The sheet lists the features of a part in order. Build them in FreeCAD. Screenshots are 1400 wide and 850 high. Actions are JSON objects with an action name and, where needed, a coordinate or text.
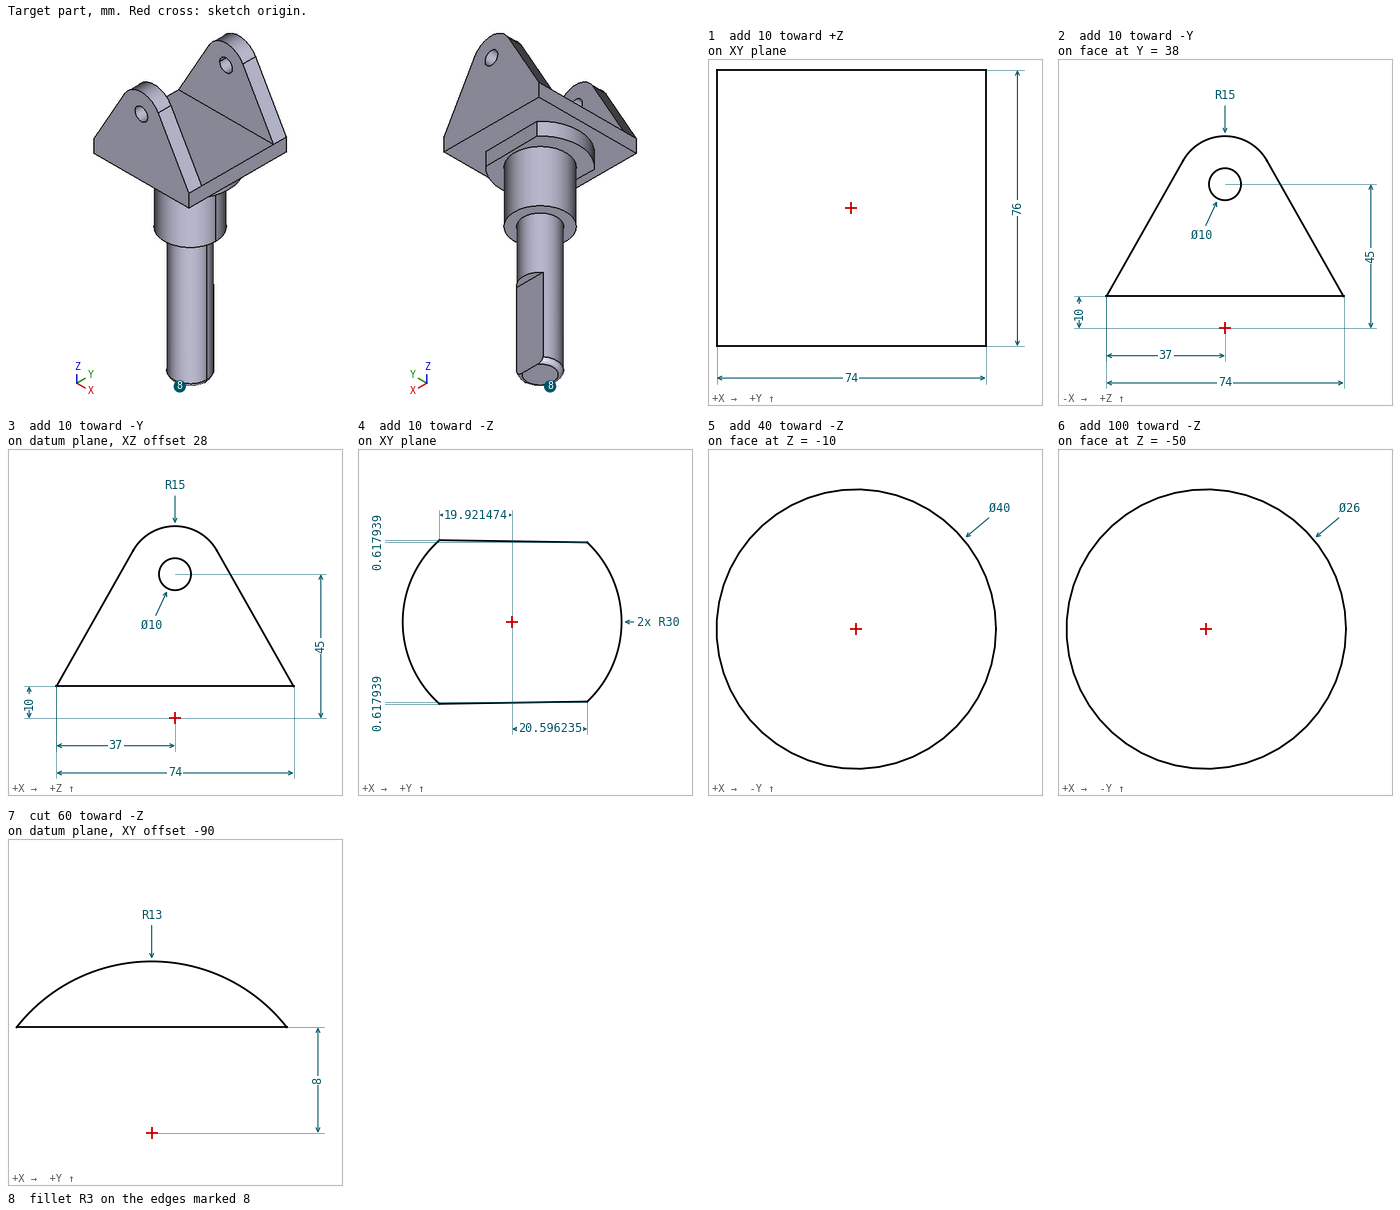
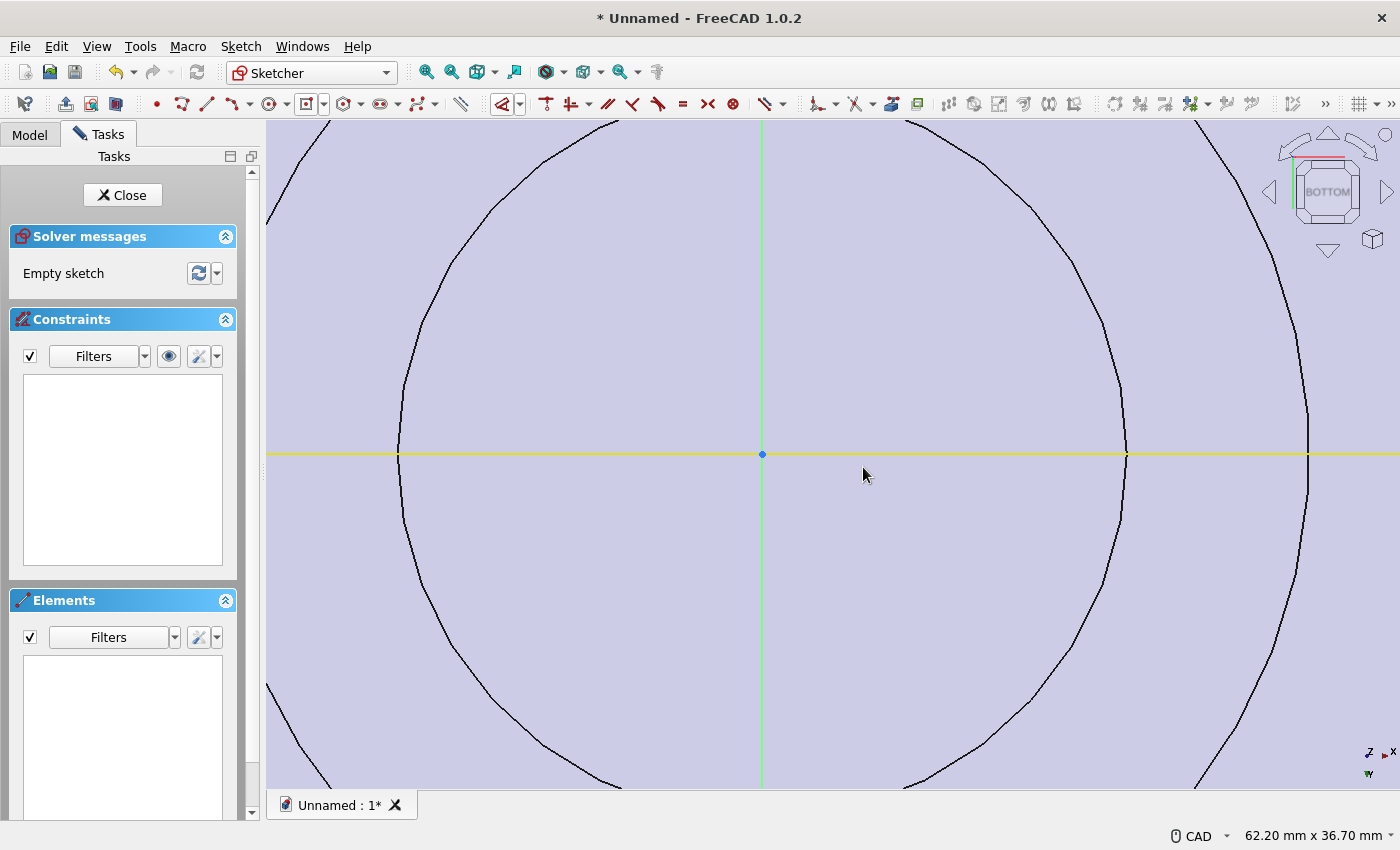
{"action": "left_click", "coordinate": [268, 104]}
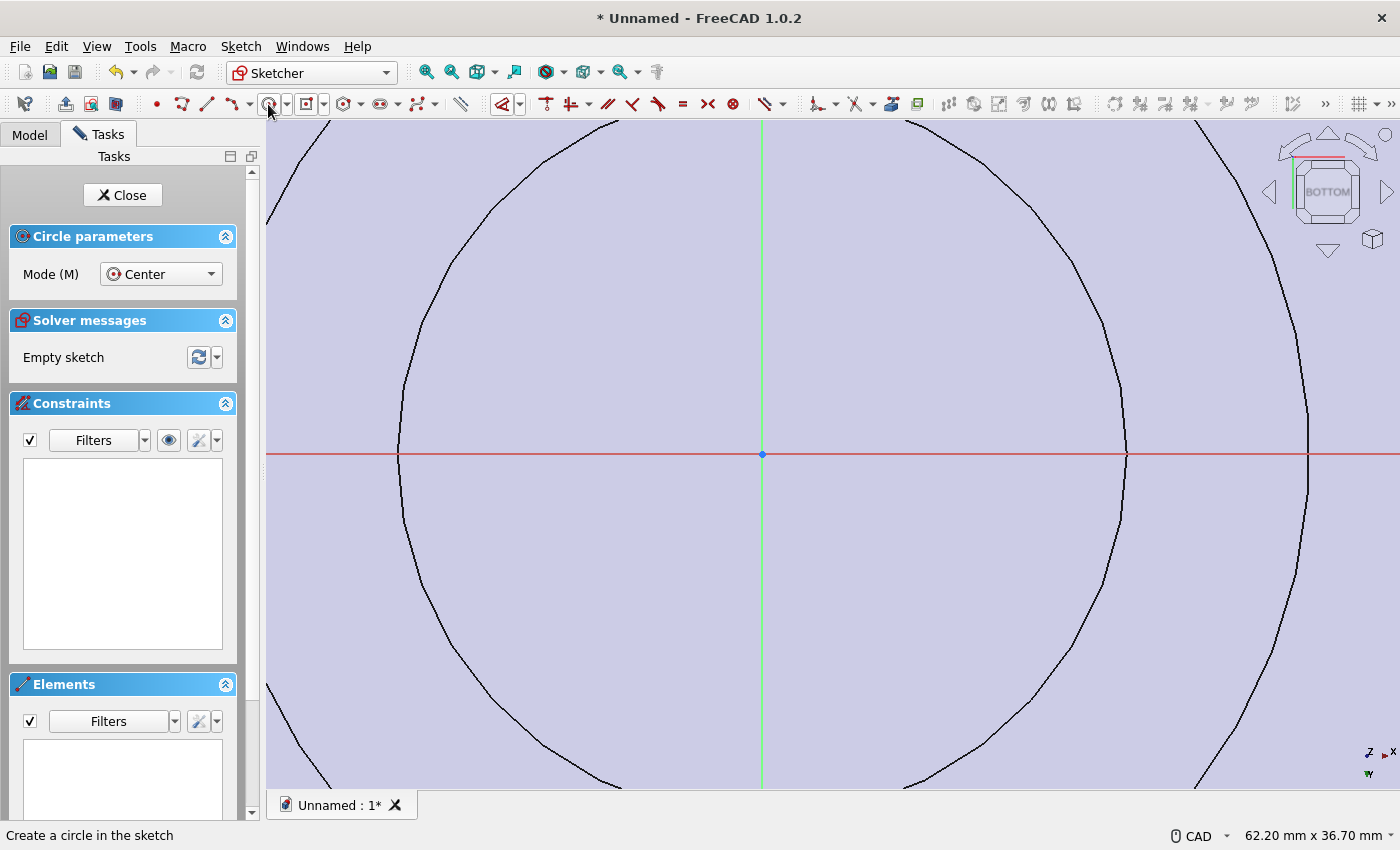
{"action": "left_click", "coordinate": [762, 454]}
{"action": "left_click", "coordinate": [930, 286]}
{"action": "key", "text": "Escape"}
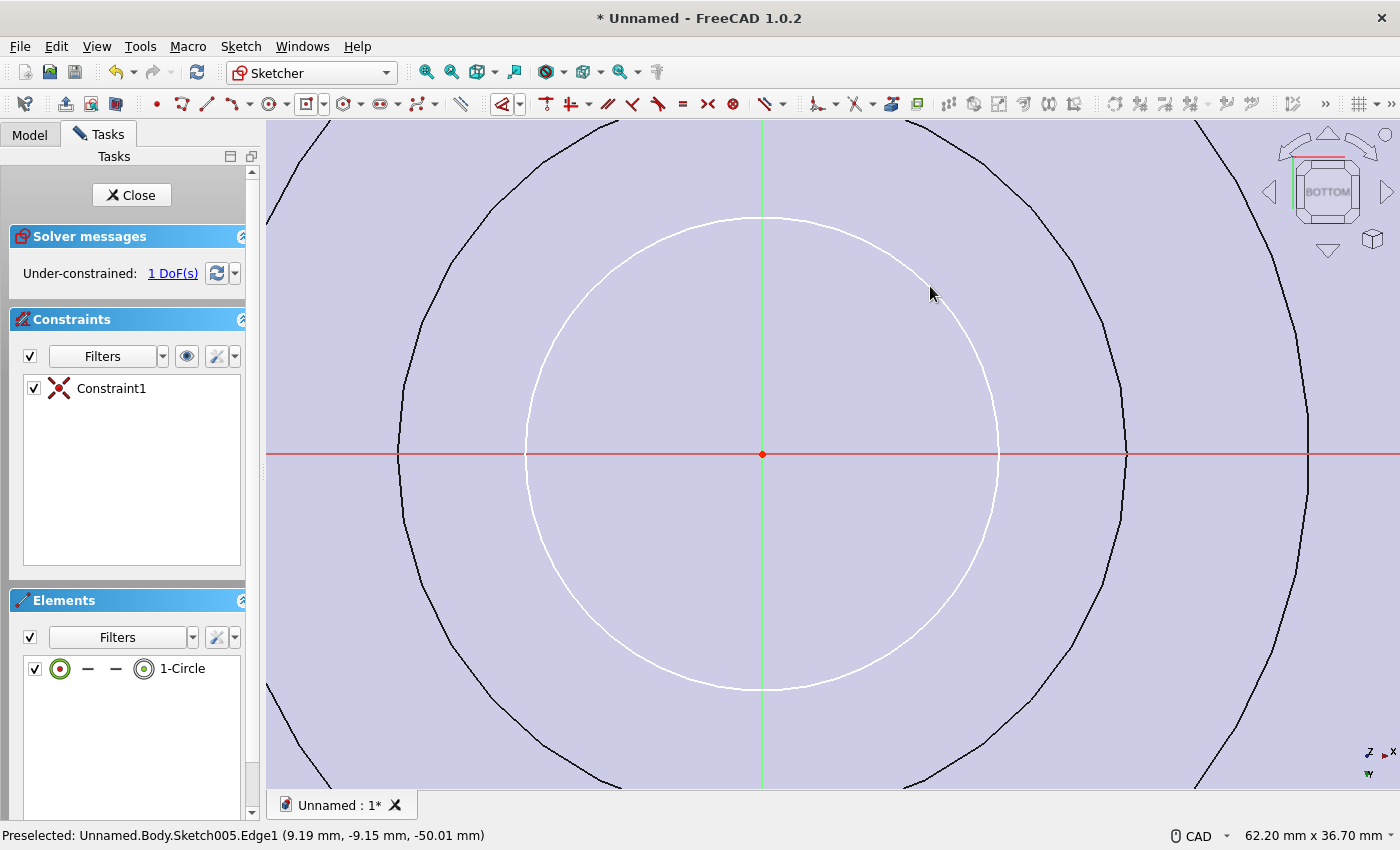
{"action": "left_click", "coordinate": [929, 286]}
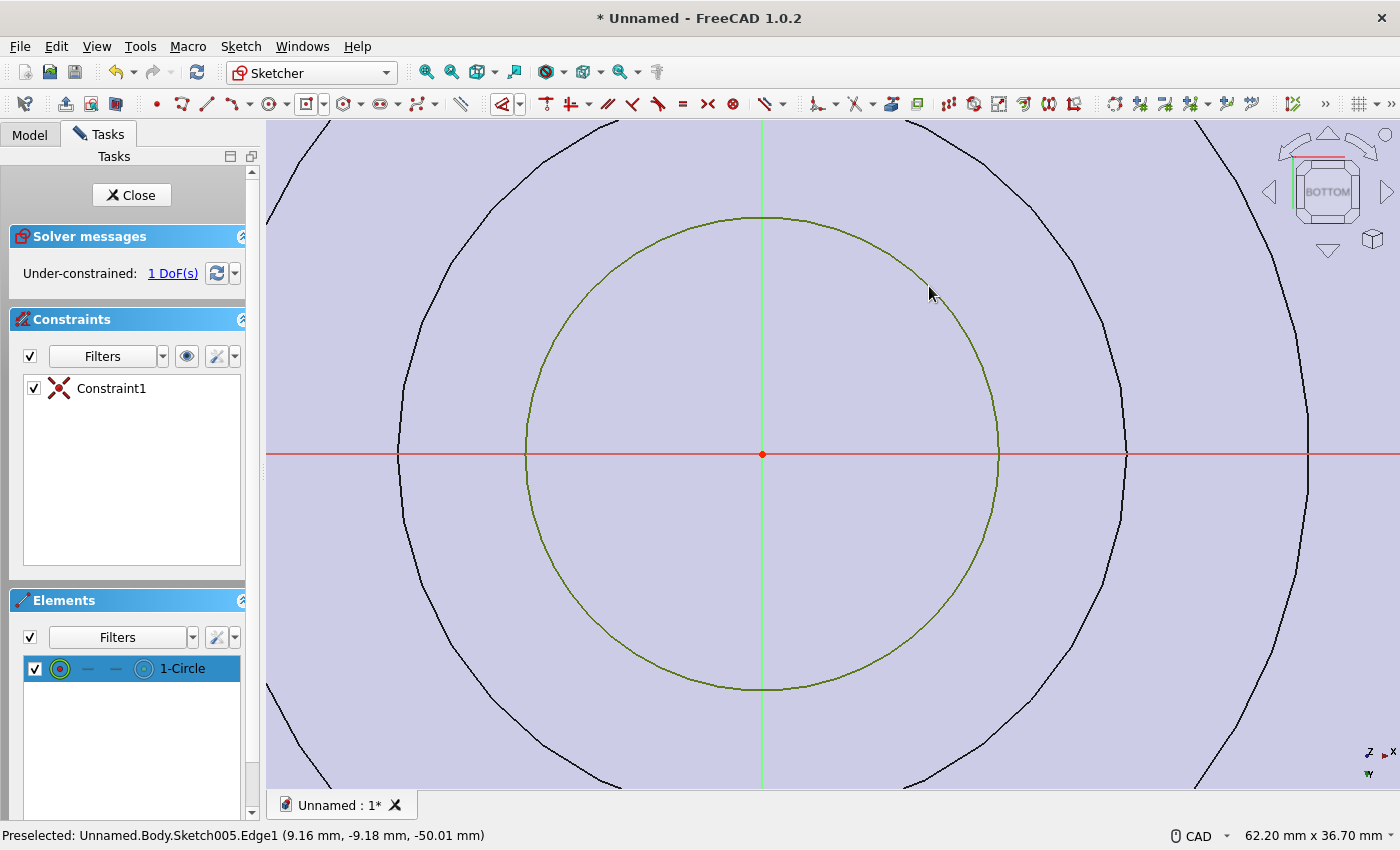
{"action": "key", "text": "k o"}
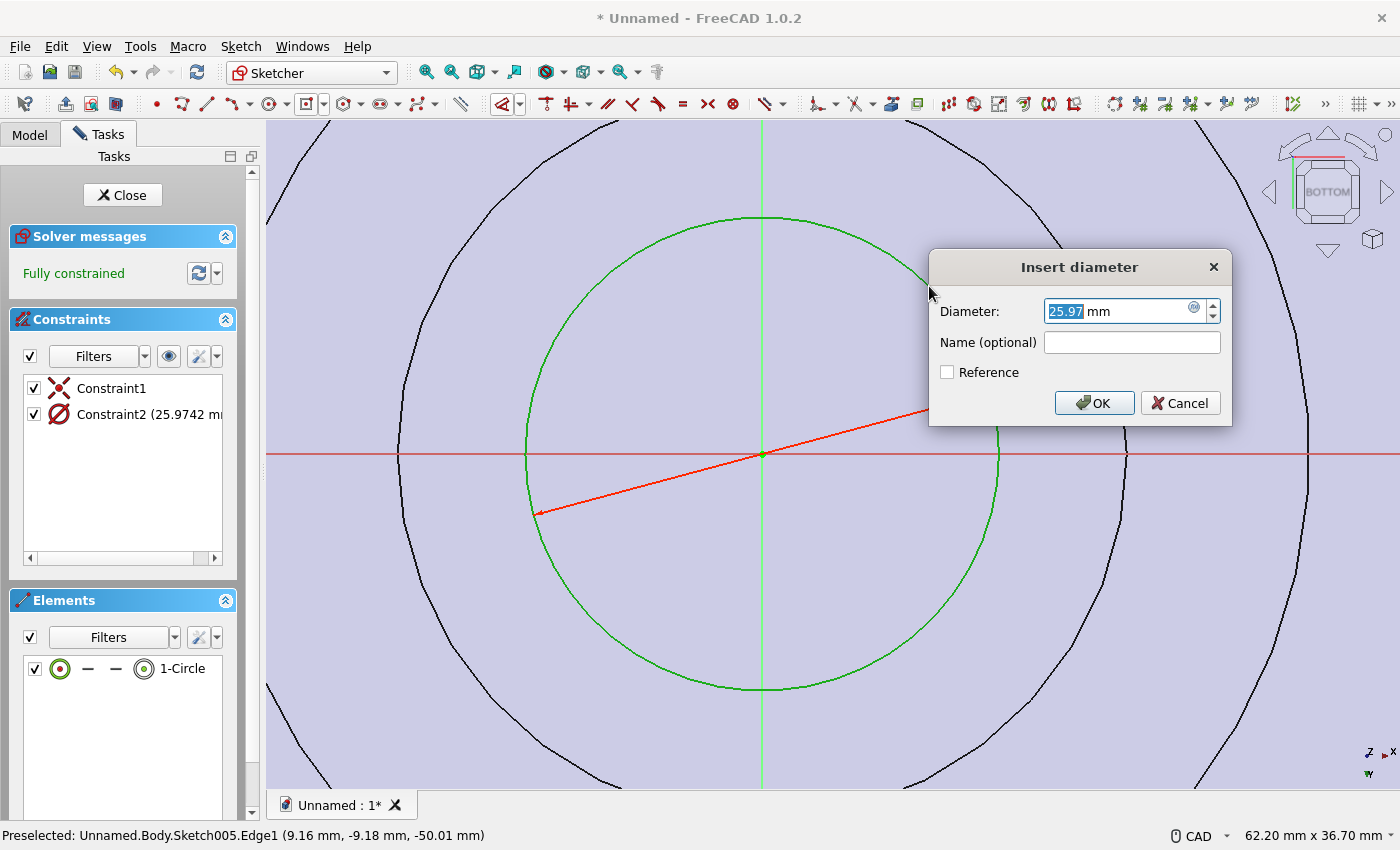
{"action": "type", "text": "26"}
{"action": "key", "text": "Return"}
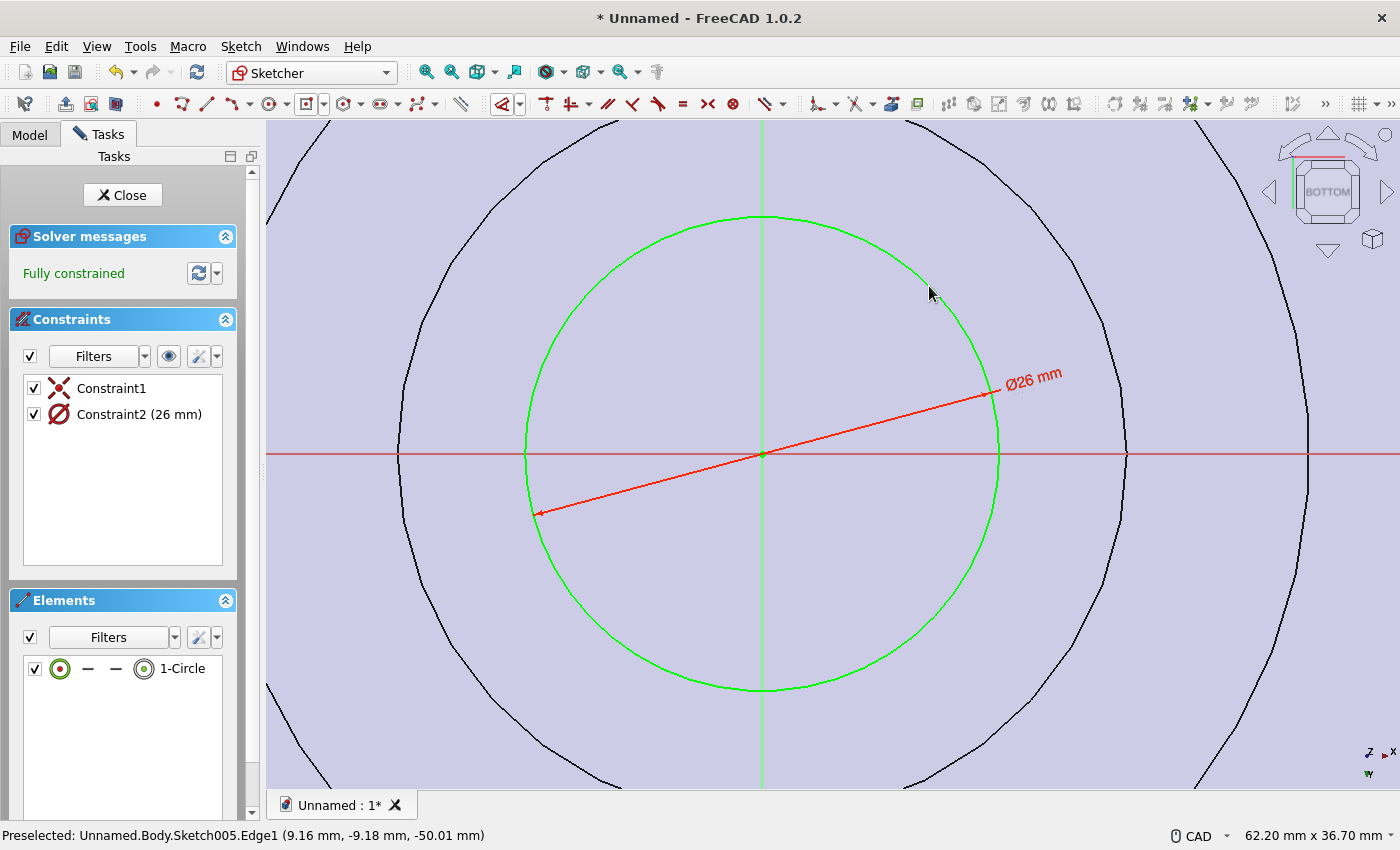
{"action": "left_click", "coordinate": [123, 195]}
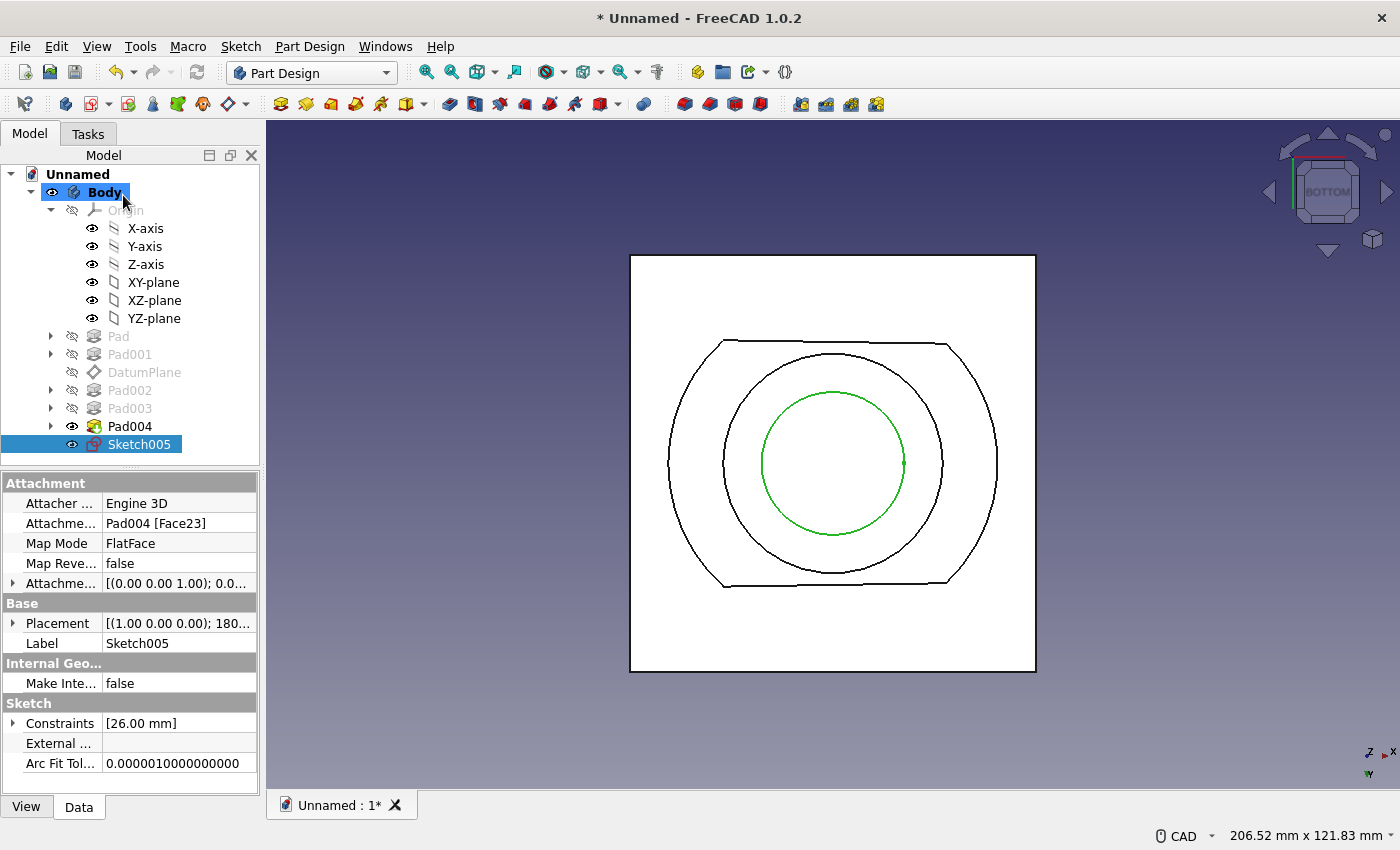
{"action": "left_click", "coordinate": [281, 104]}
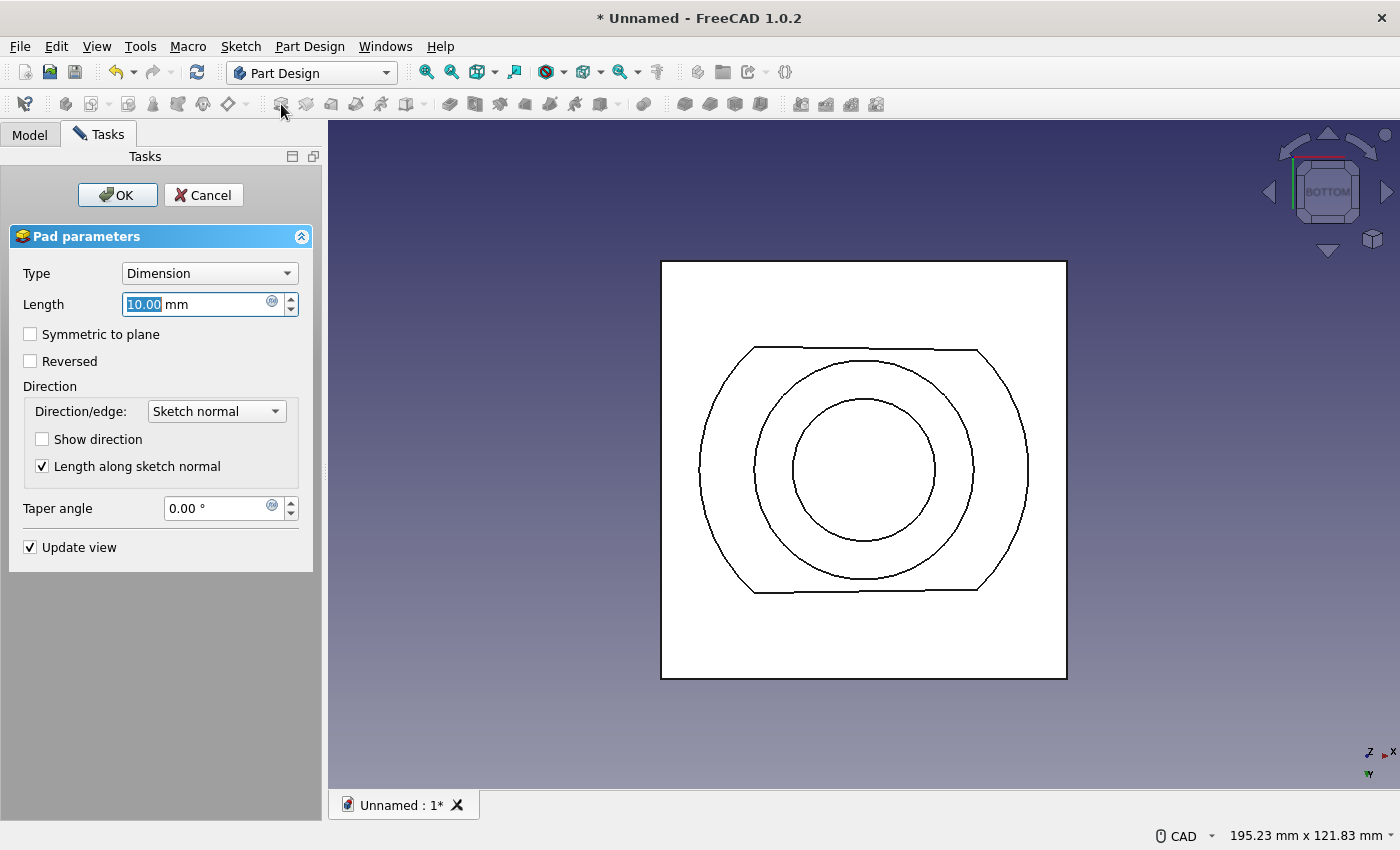
{"action": "type", "text": "100"}
{"action": "key", "text": "Tab"}